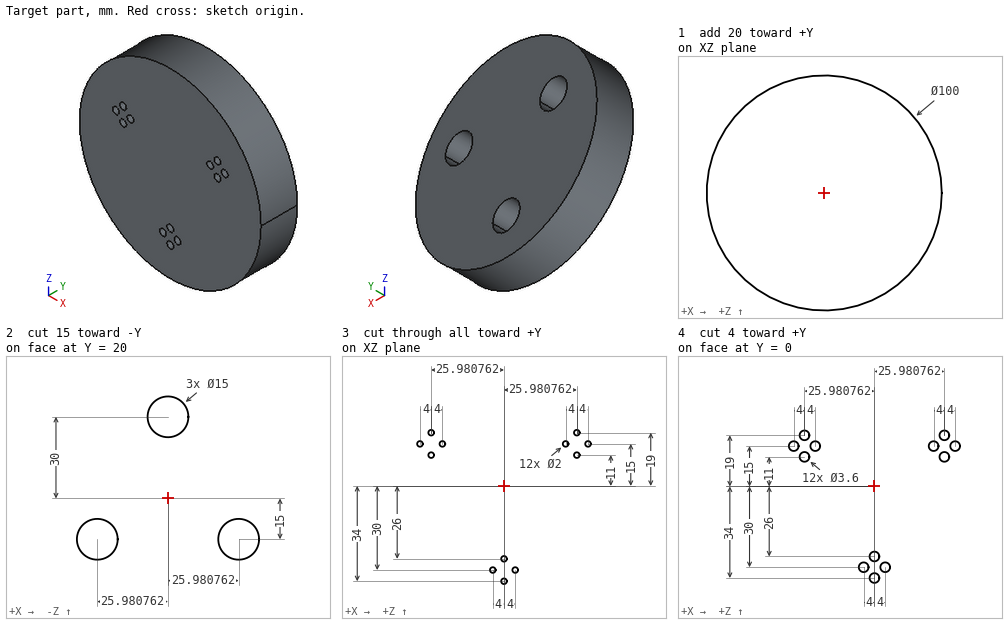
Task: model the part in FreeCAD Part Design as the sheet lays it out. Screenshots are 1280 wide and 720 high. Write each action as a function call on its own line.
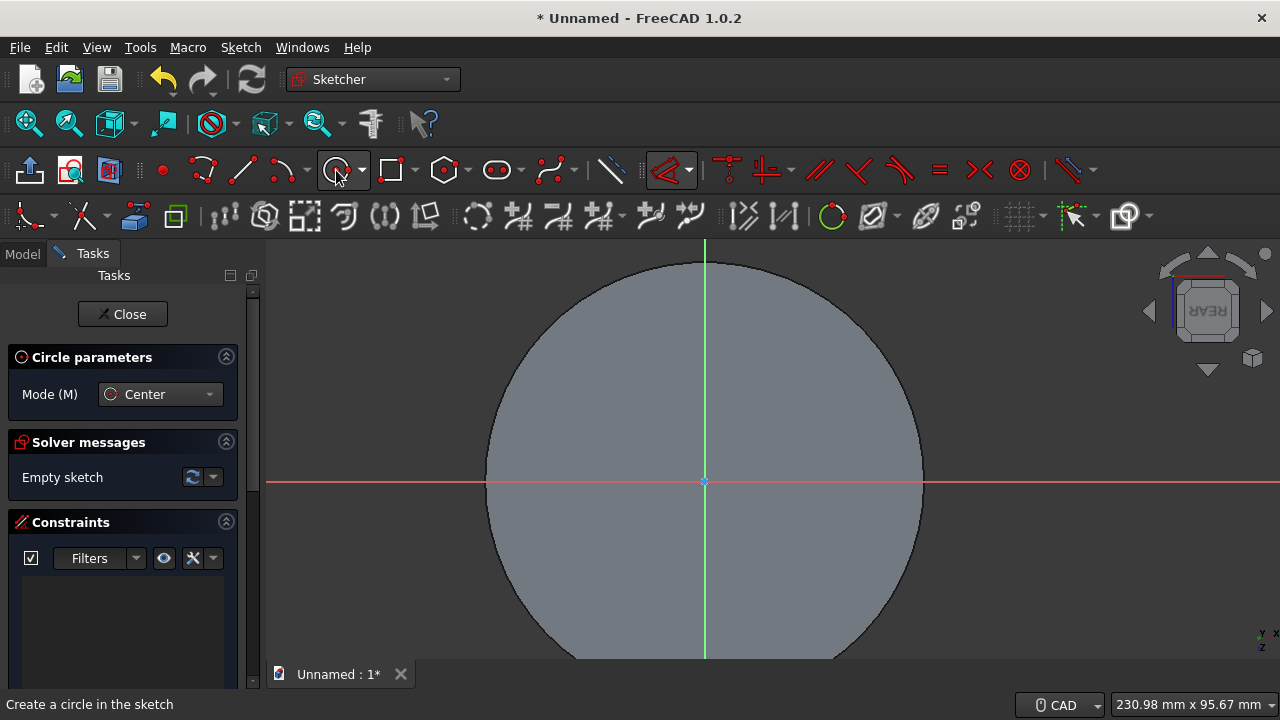
click(705, 350)
click(728, 327)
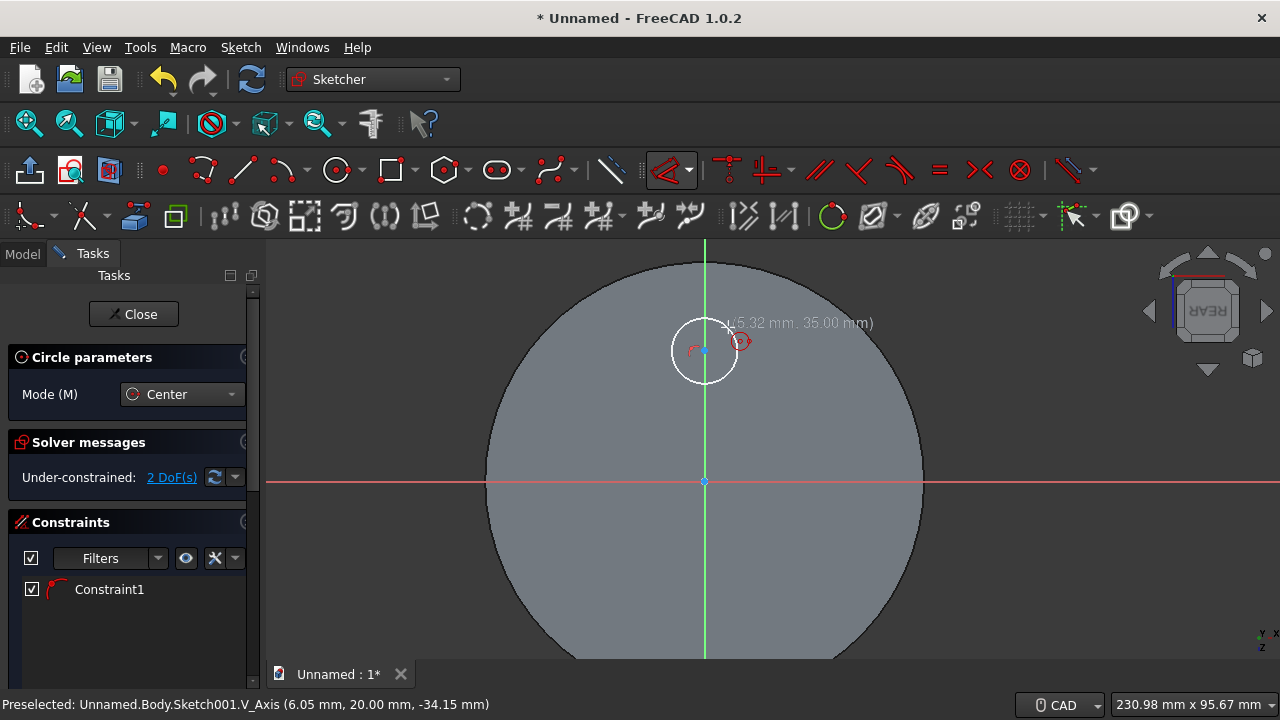
click(819, 547)
click(842, 524)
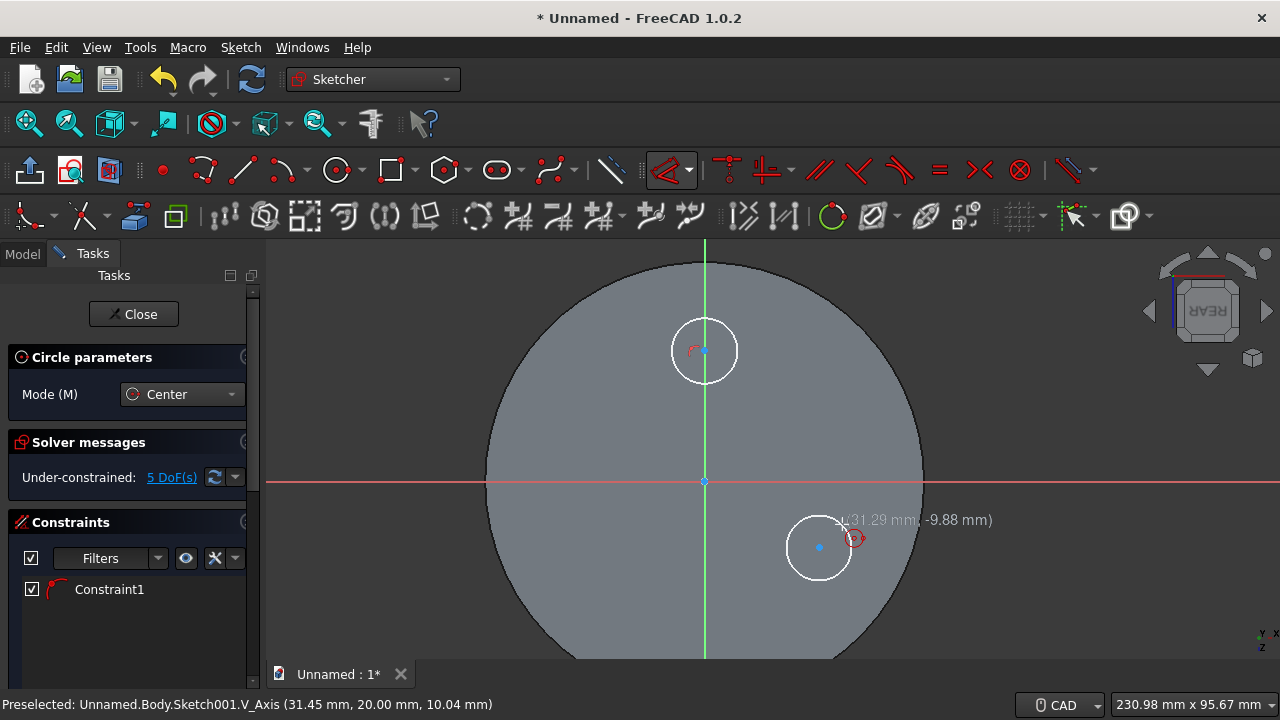
click(591, 547)
click(614, 524)
key(Escape)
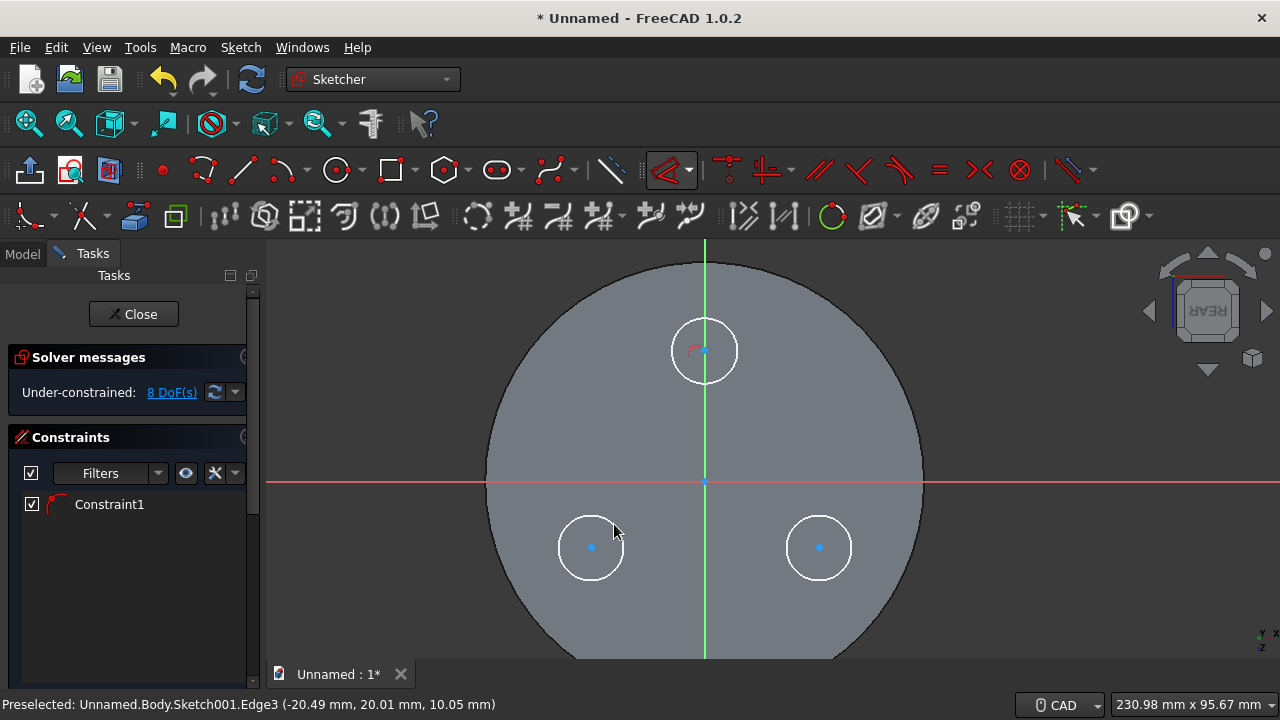
click(728, 328)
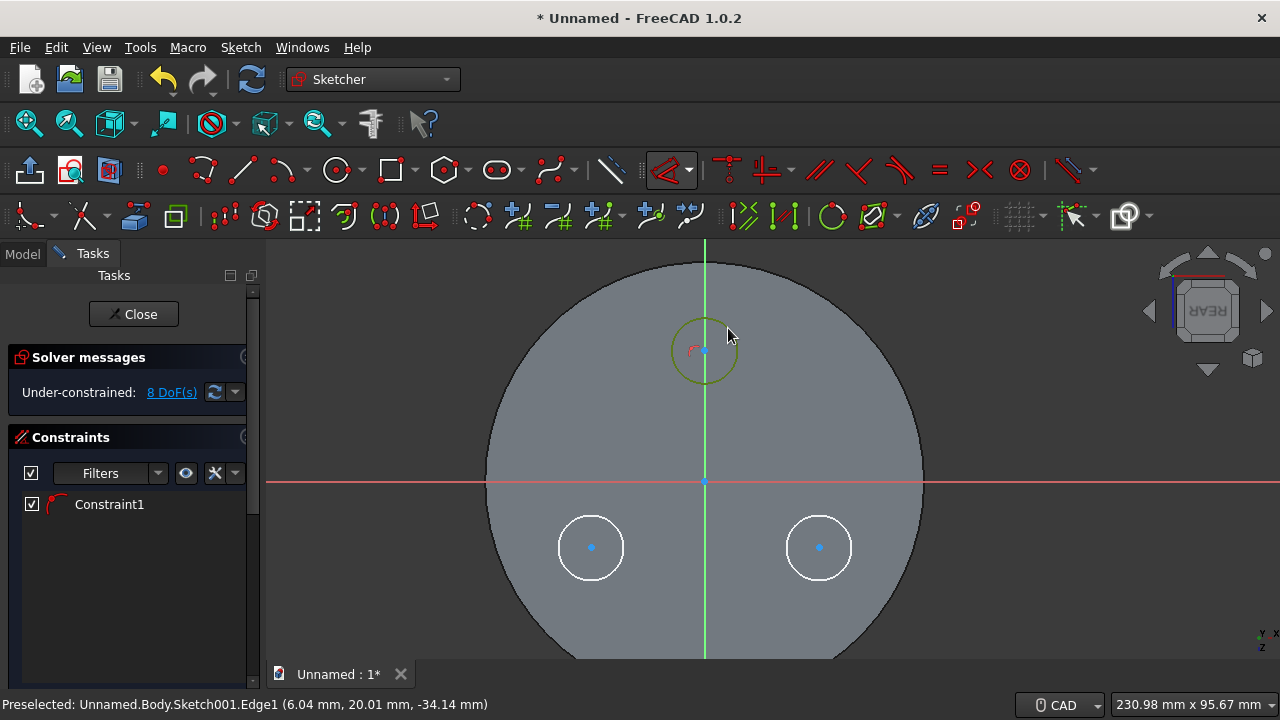
click(842, 525)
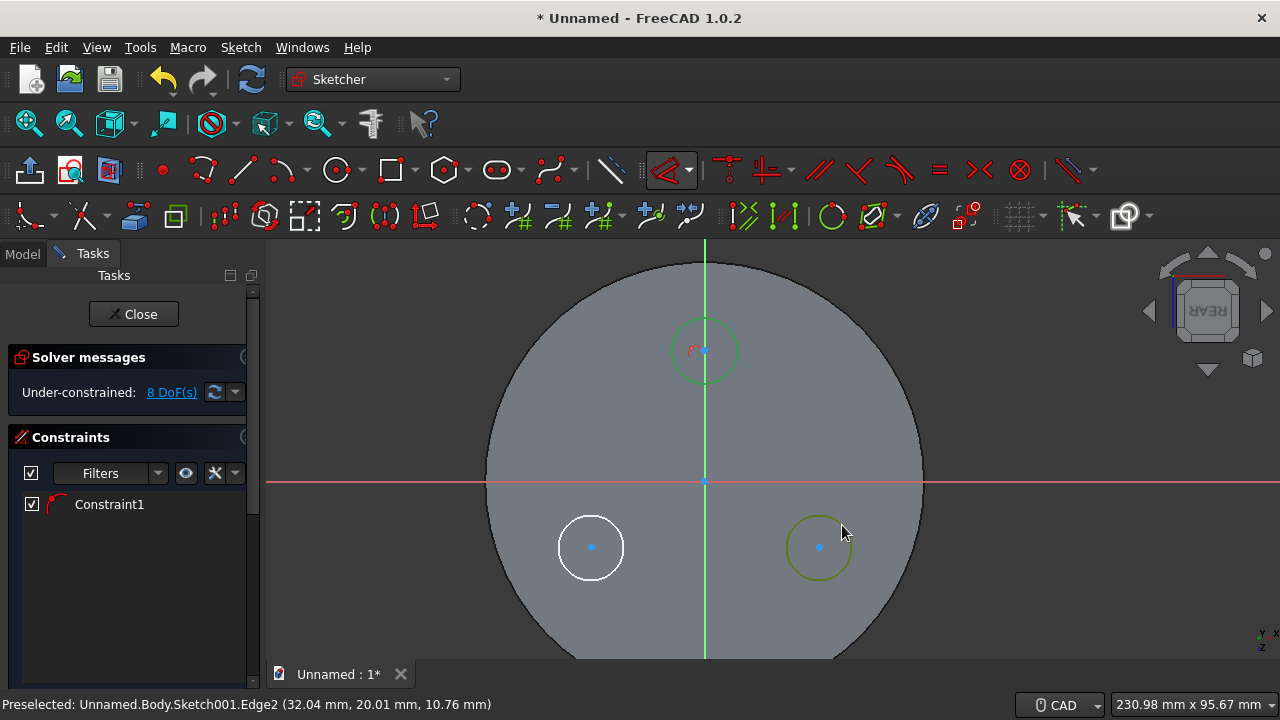
click(614, 525)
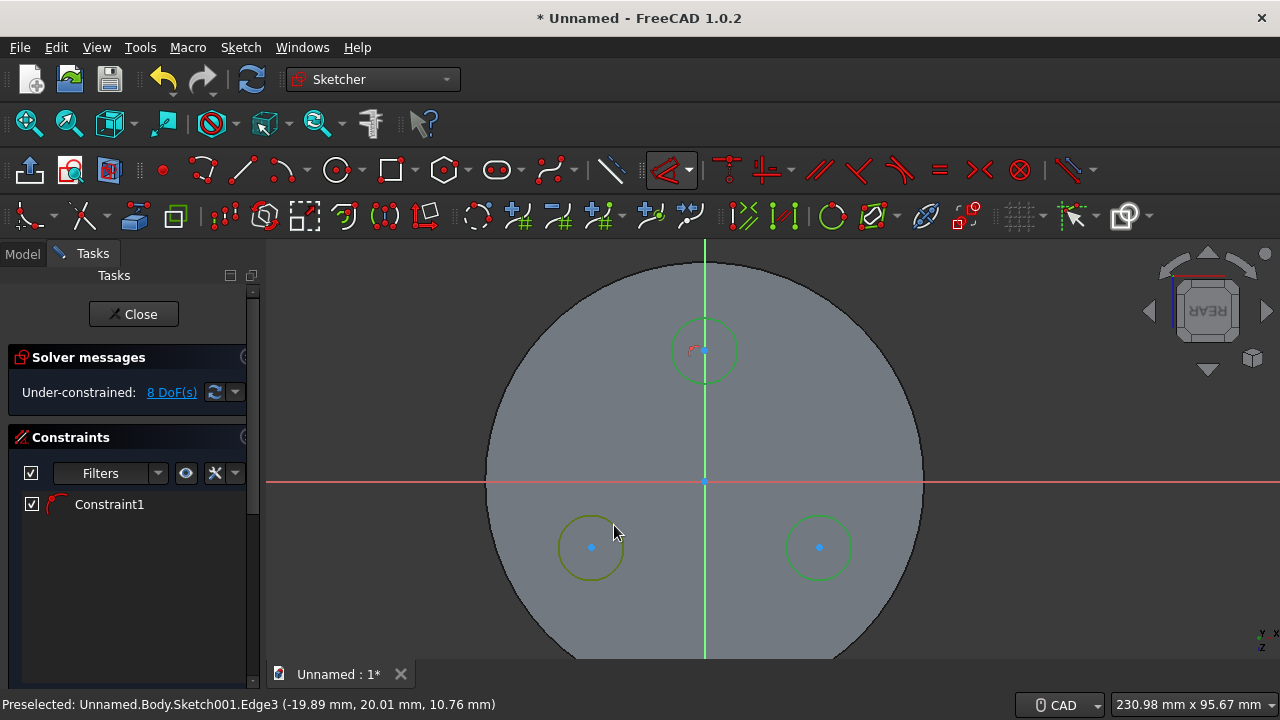
click(940, 170)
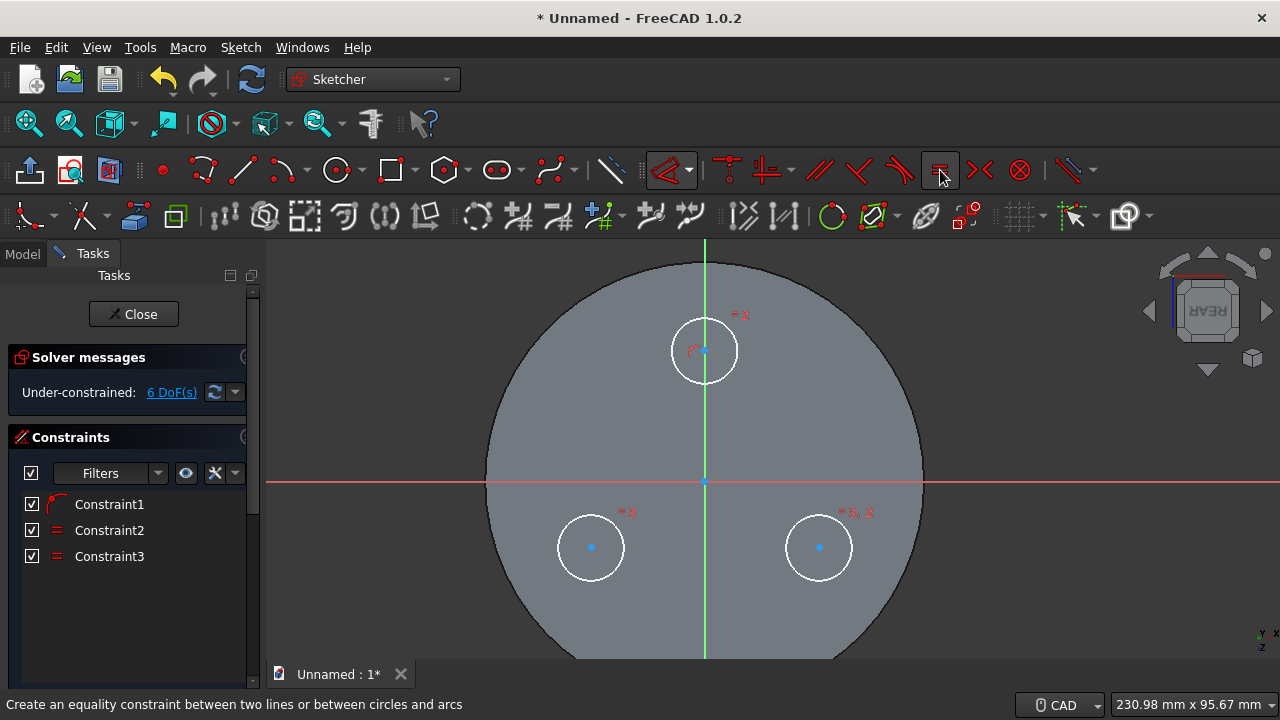
click(819, 548)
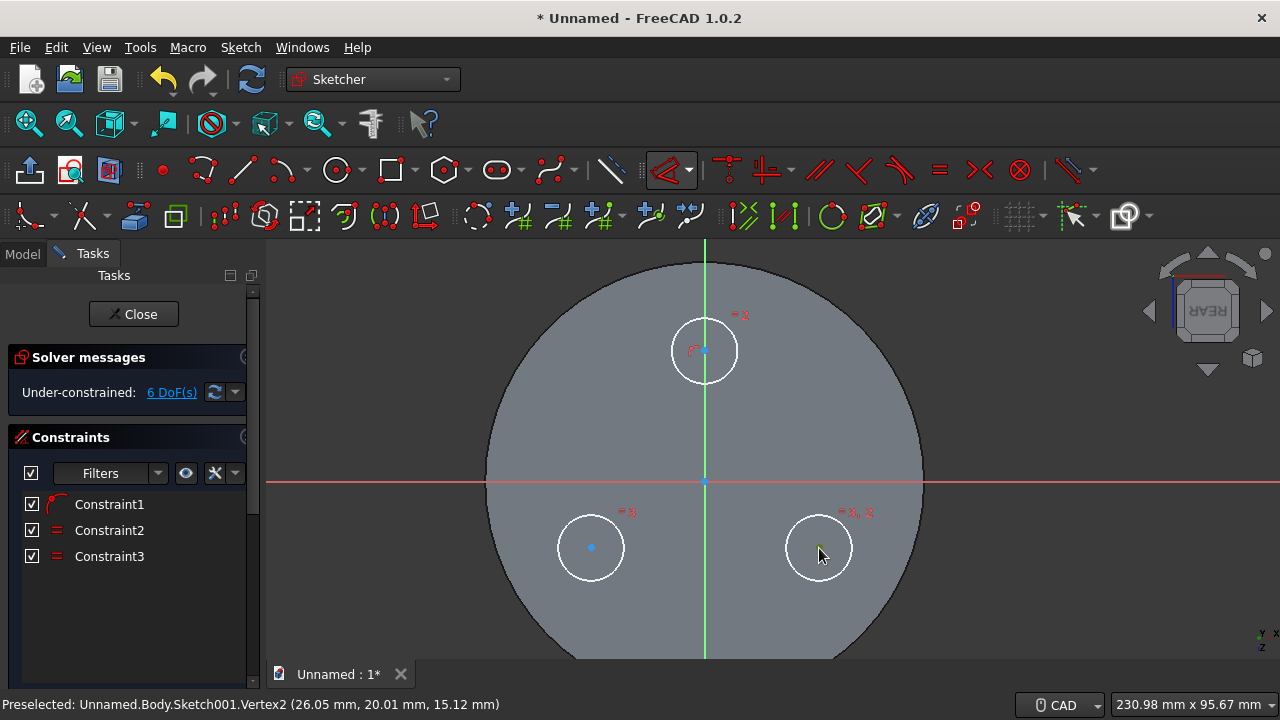
click(591, 548)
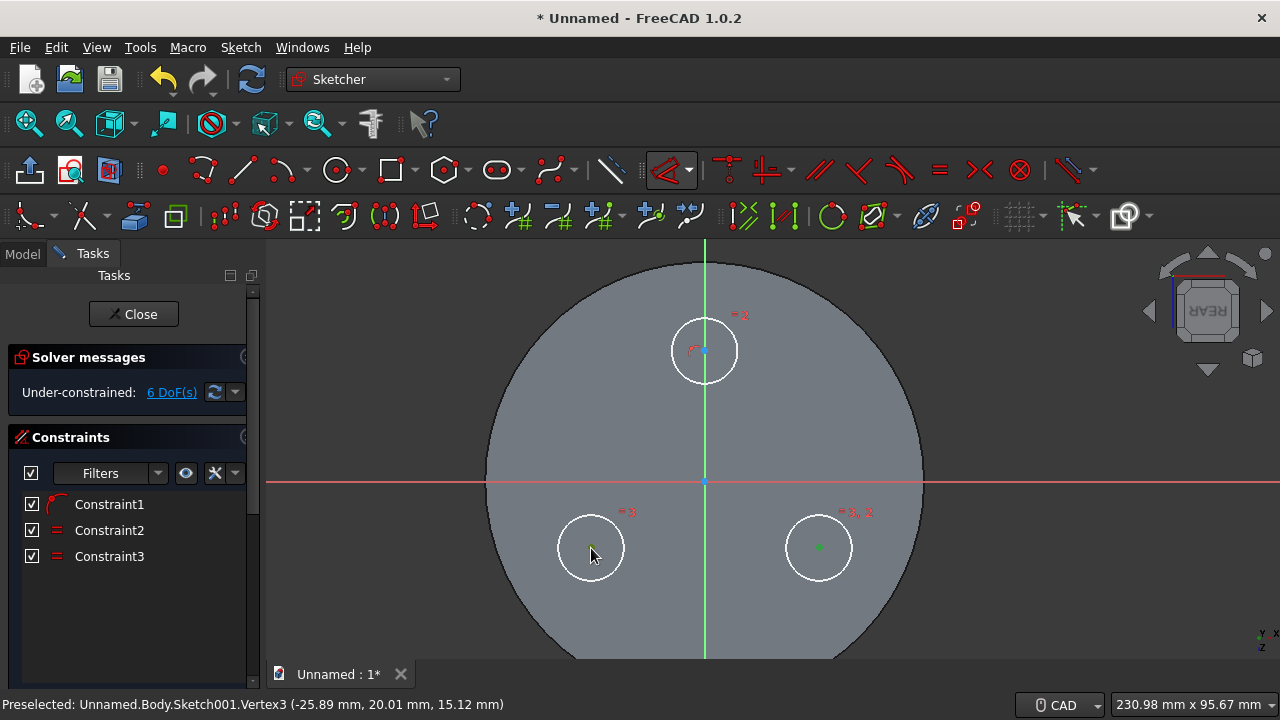
click(794, 170)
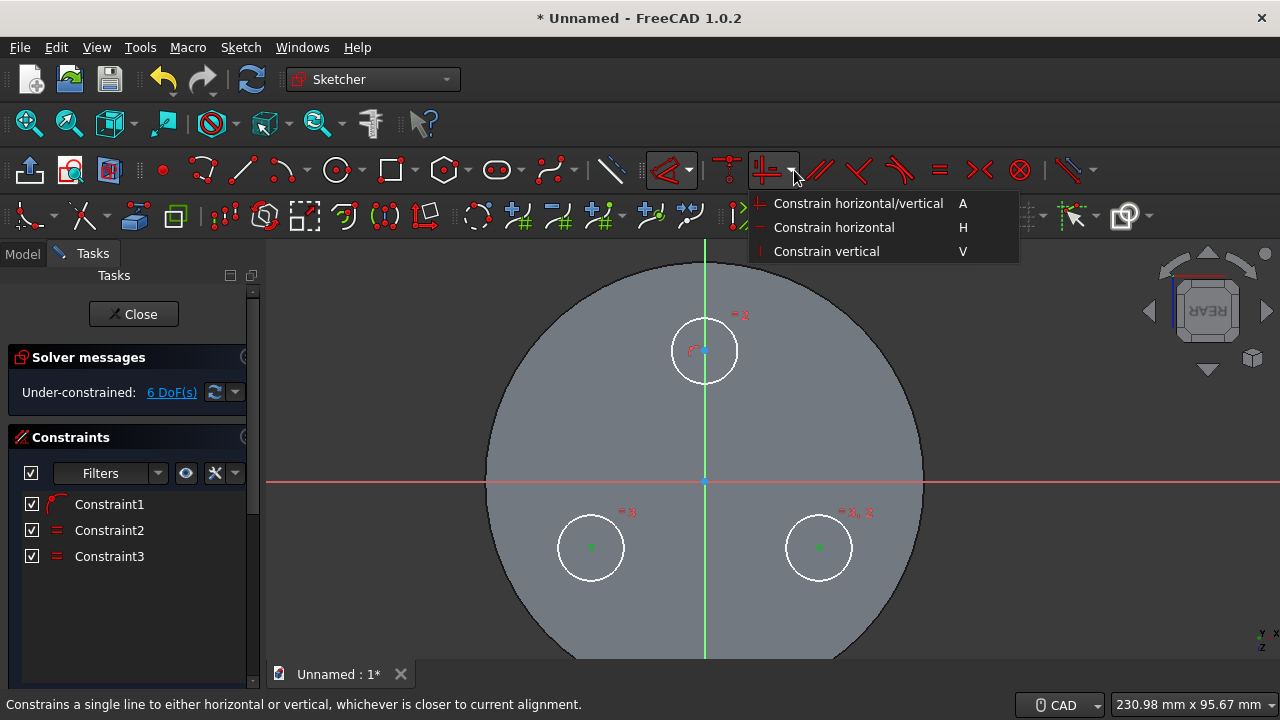
click(884, 227)